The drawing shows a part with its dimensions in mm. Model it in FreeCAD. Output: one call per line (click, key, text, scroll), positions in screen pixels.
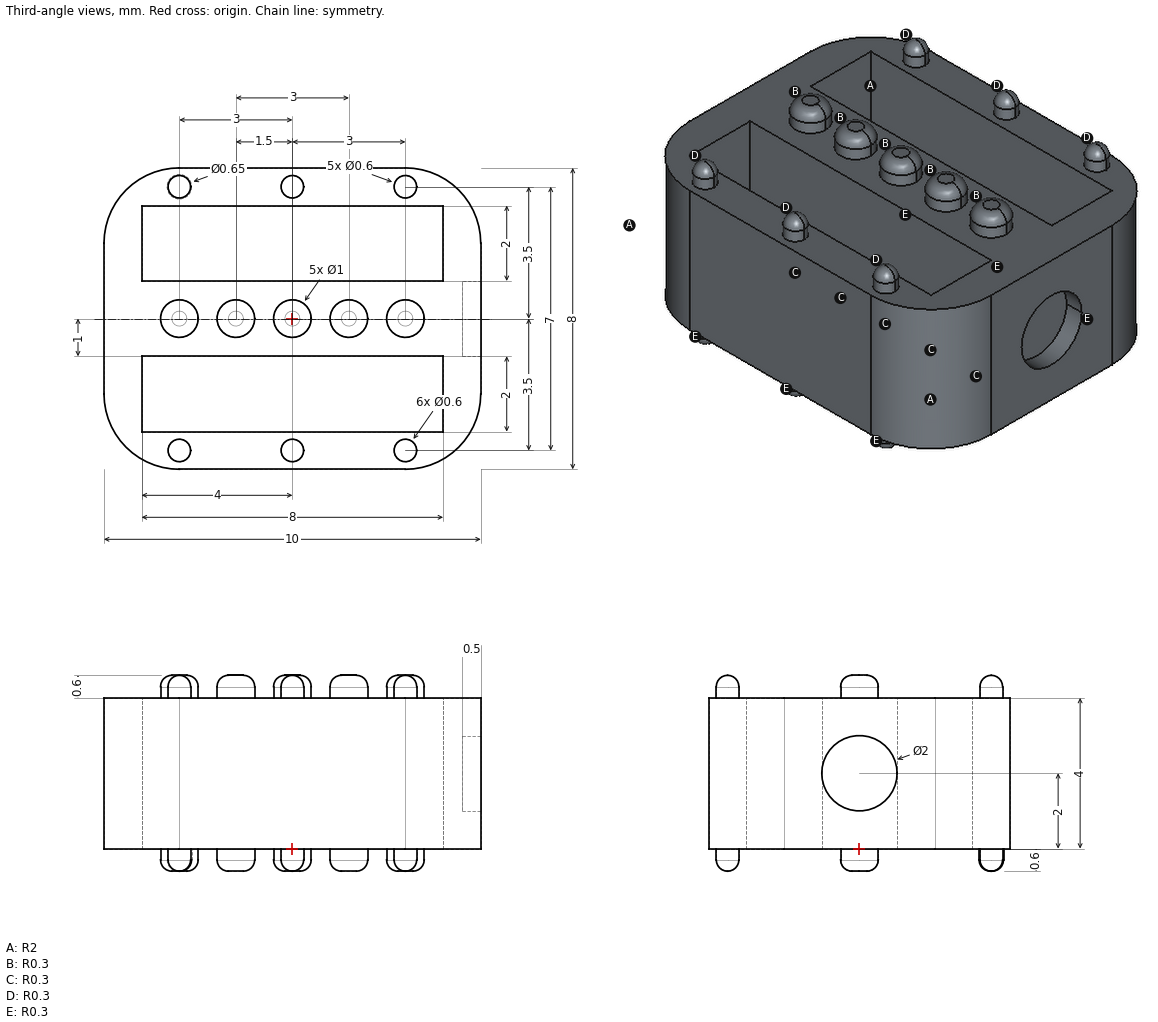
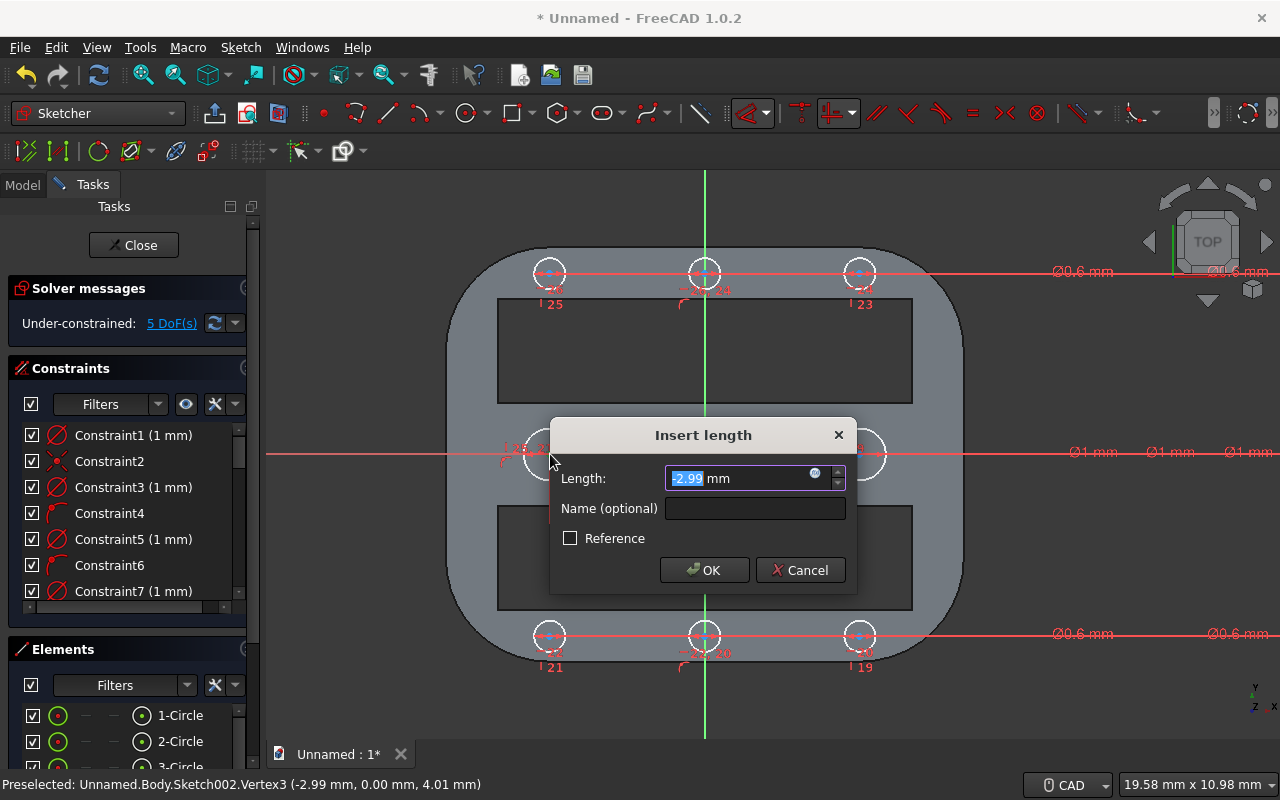
text(-3)
key(Return)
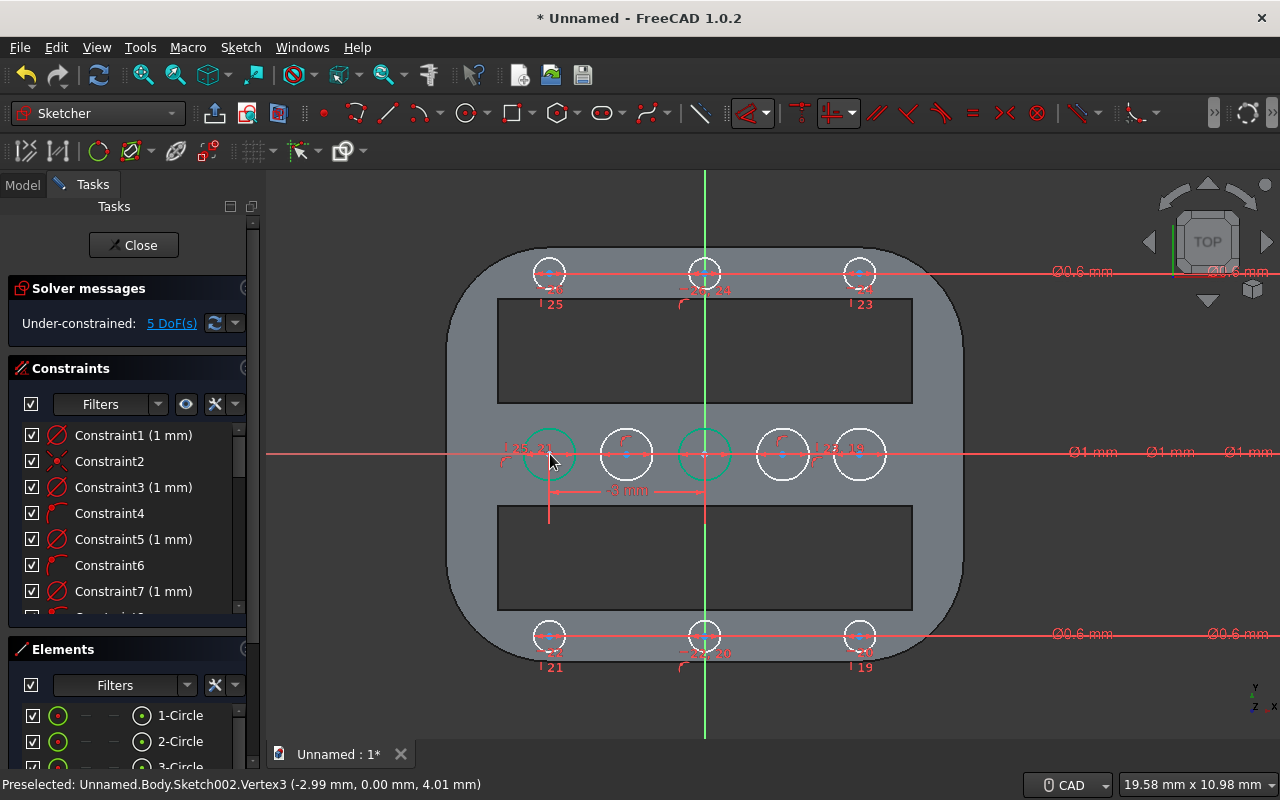
click(860, 454)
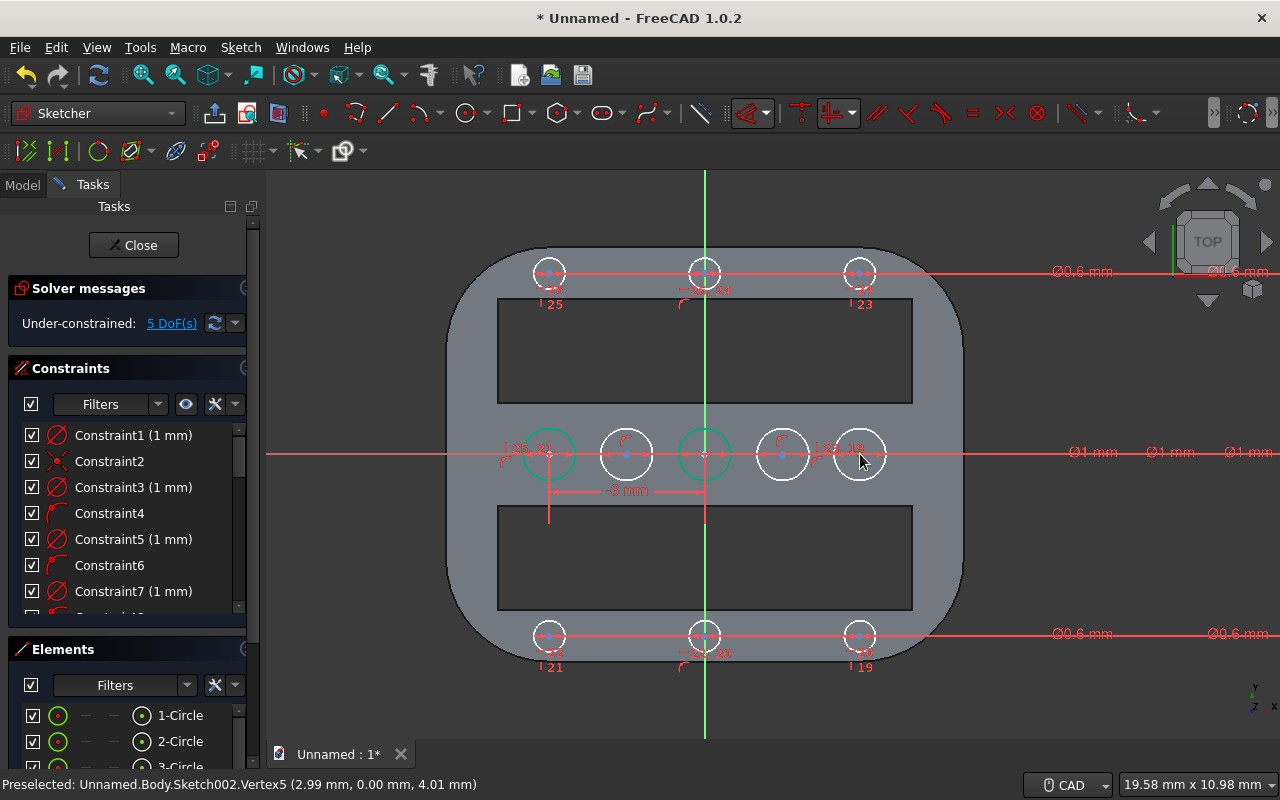
key(l)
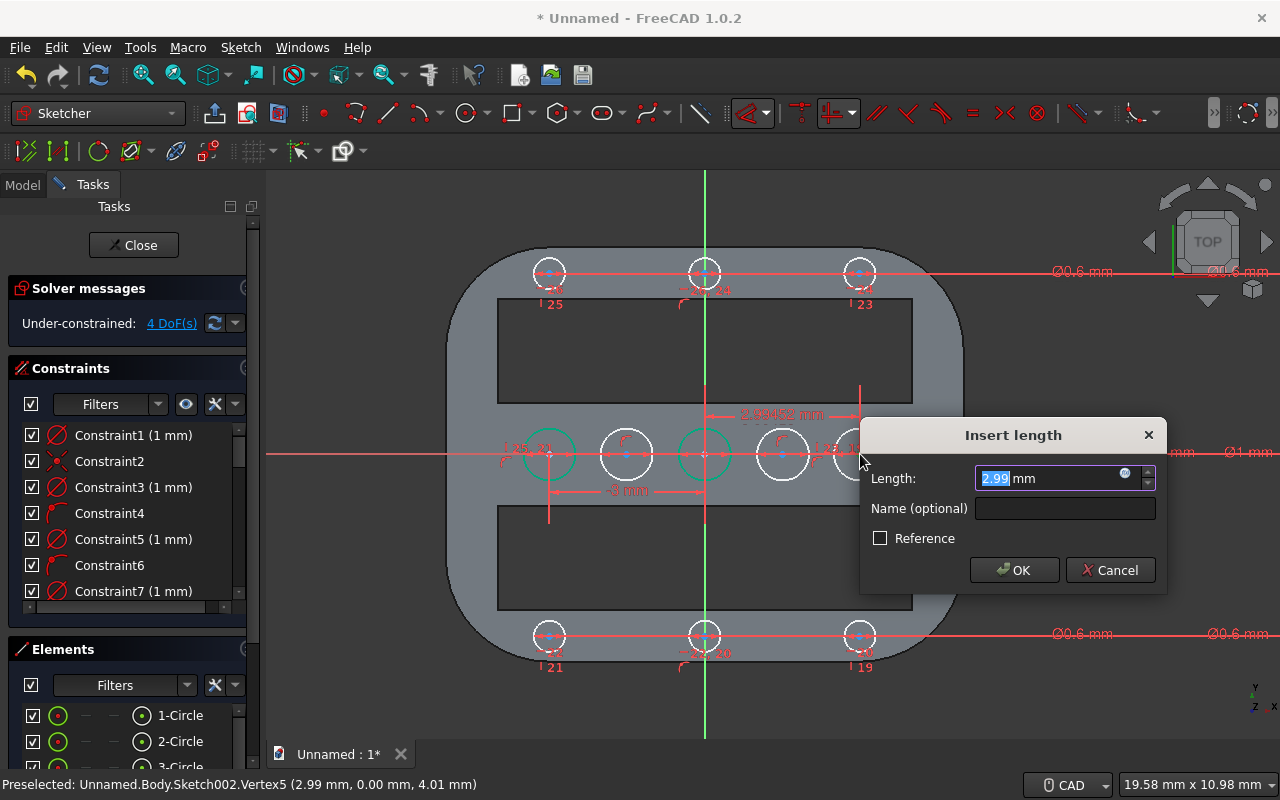
text(3)
key(Return)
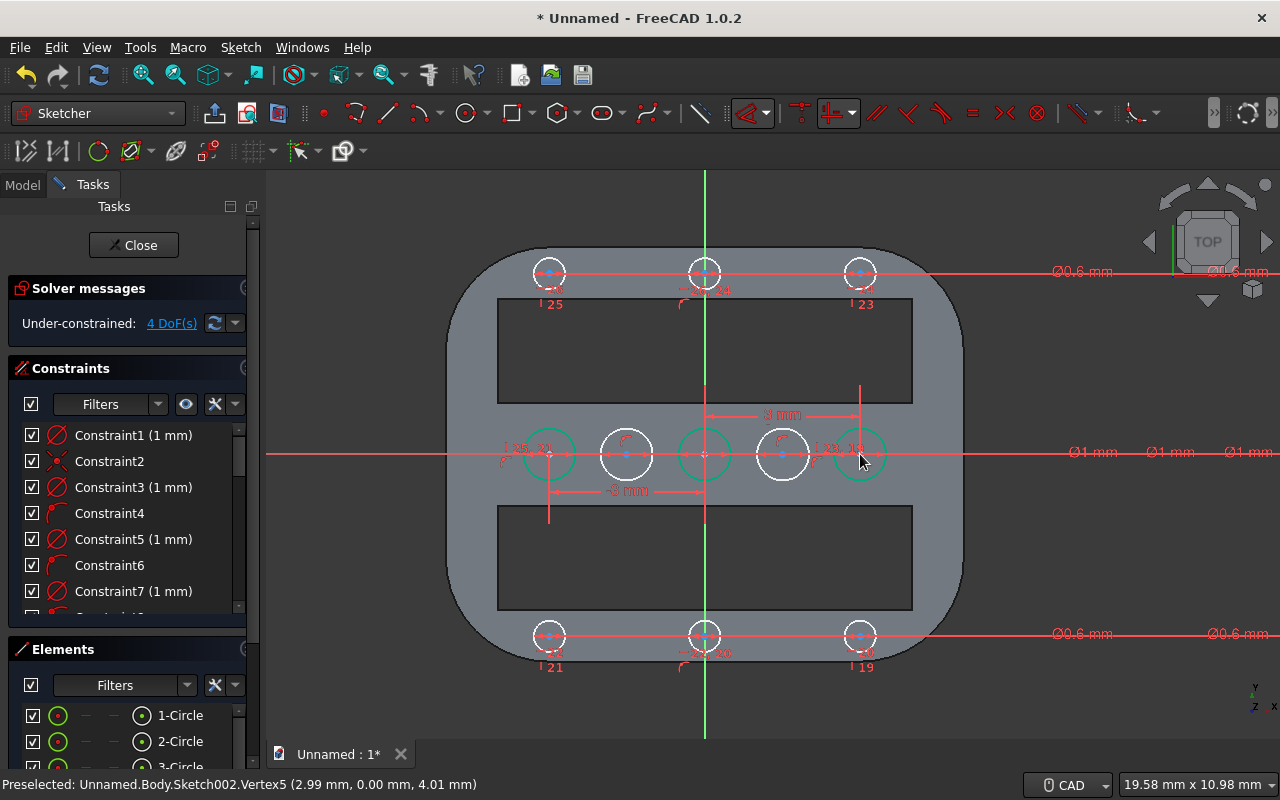
click(627, 454)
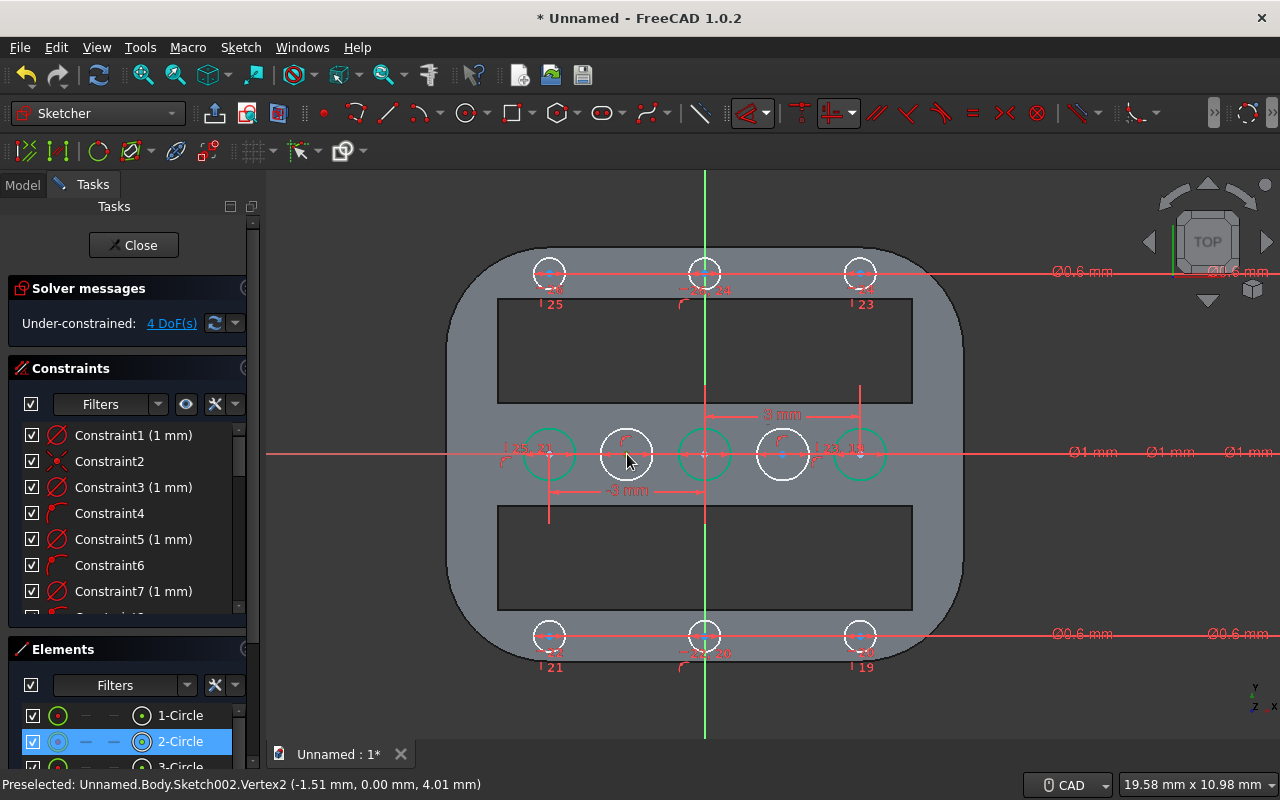
click(783, 454)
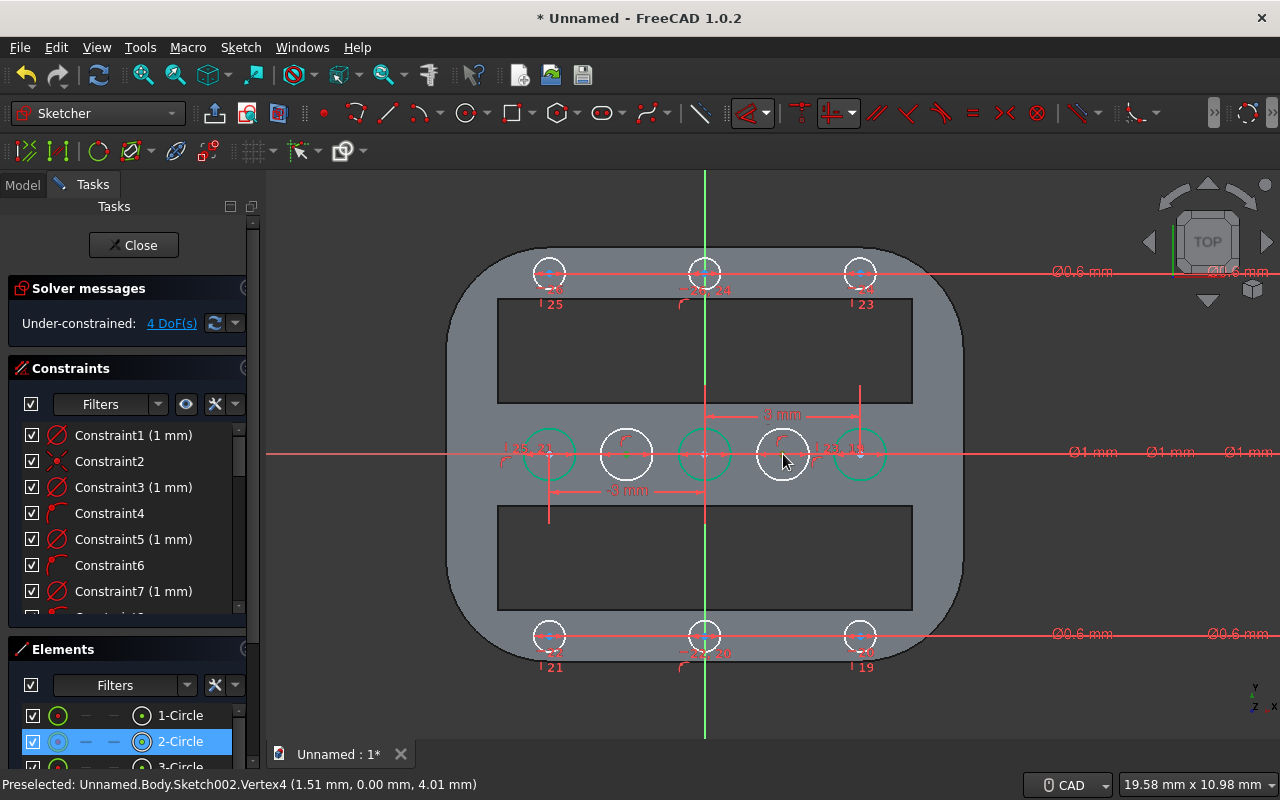
key(l)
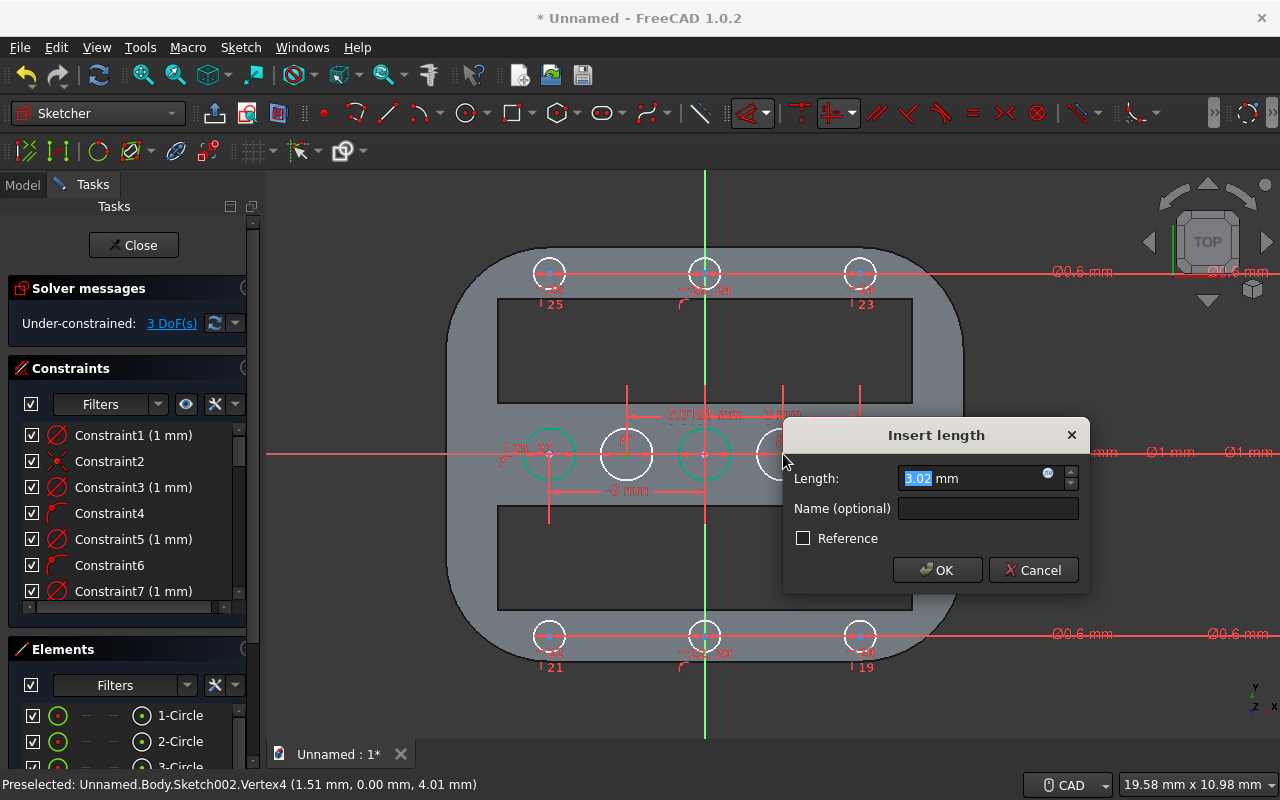
text(3)
key(Return)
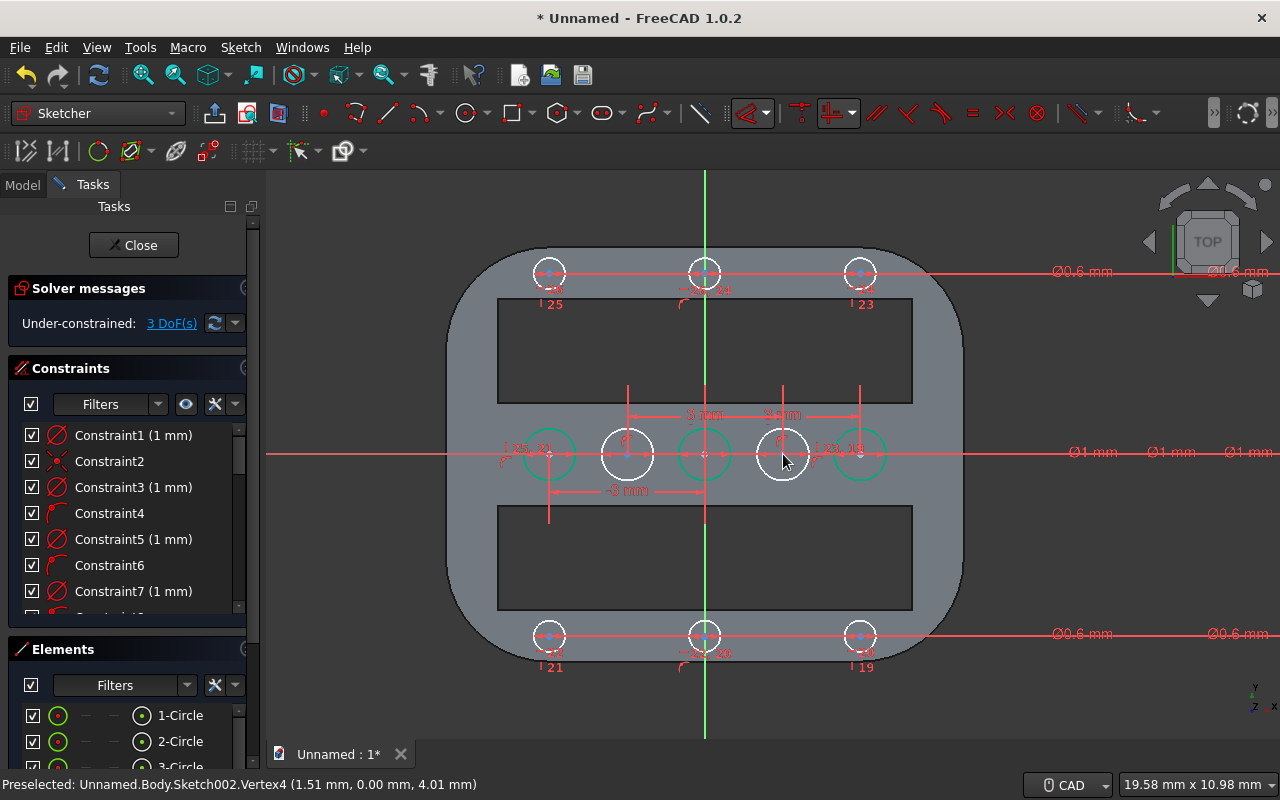
click(860, 636)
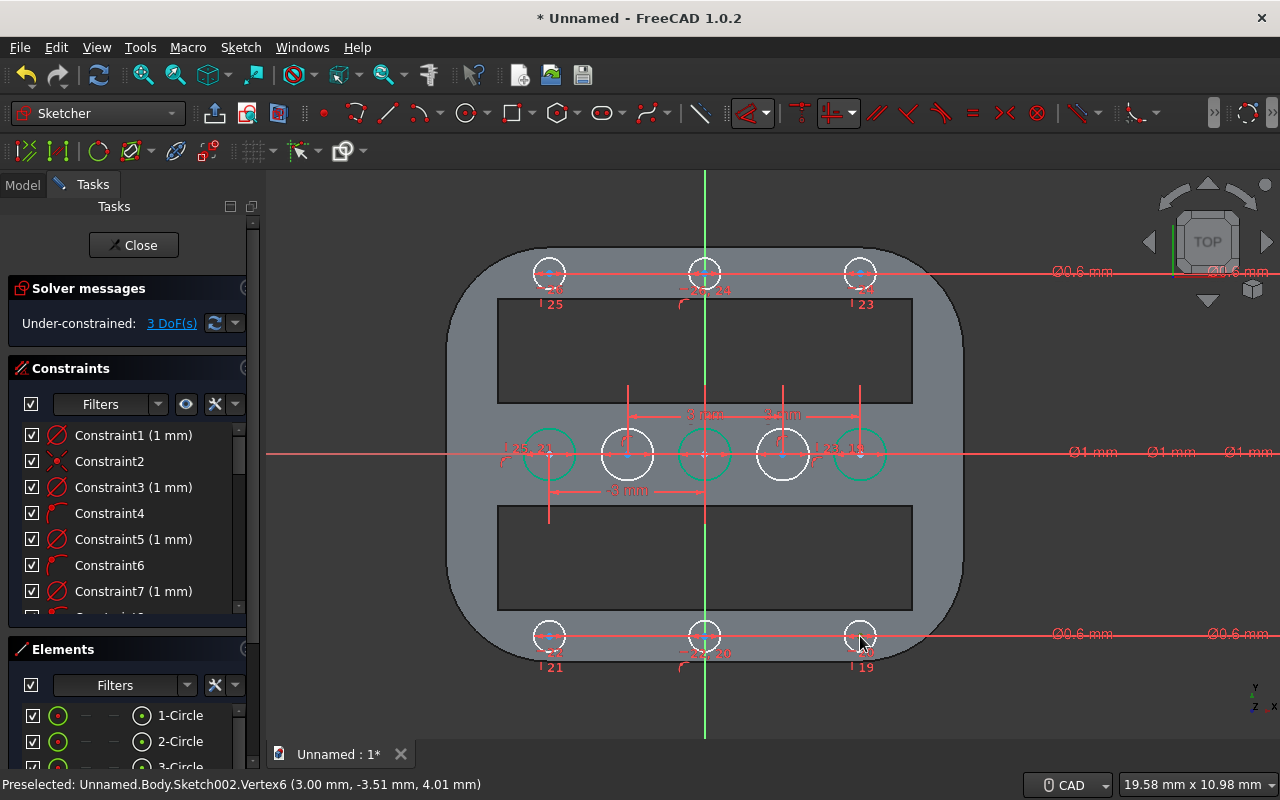
click(860, 274)